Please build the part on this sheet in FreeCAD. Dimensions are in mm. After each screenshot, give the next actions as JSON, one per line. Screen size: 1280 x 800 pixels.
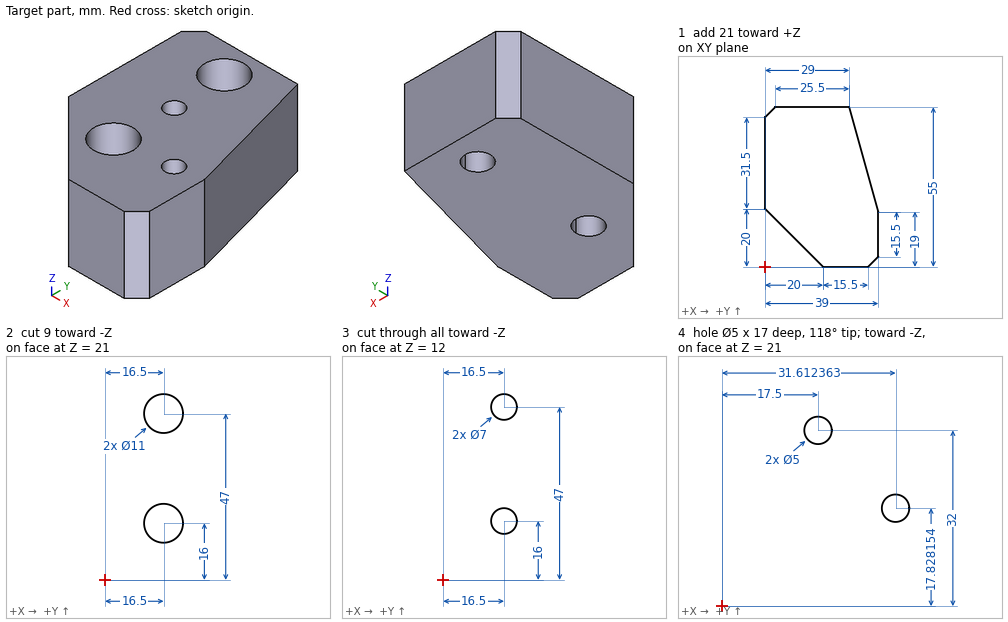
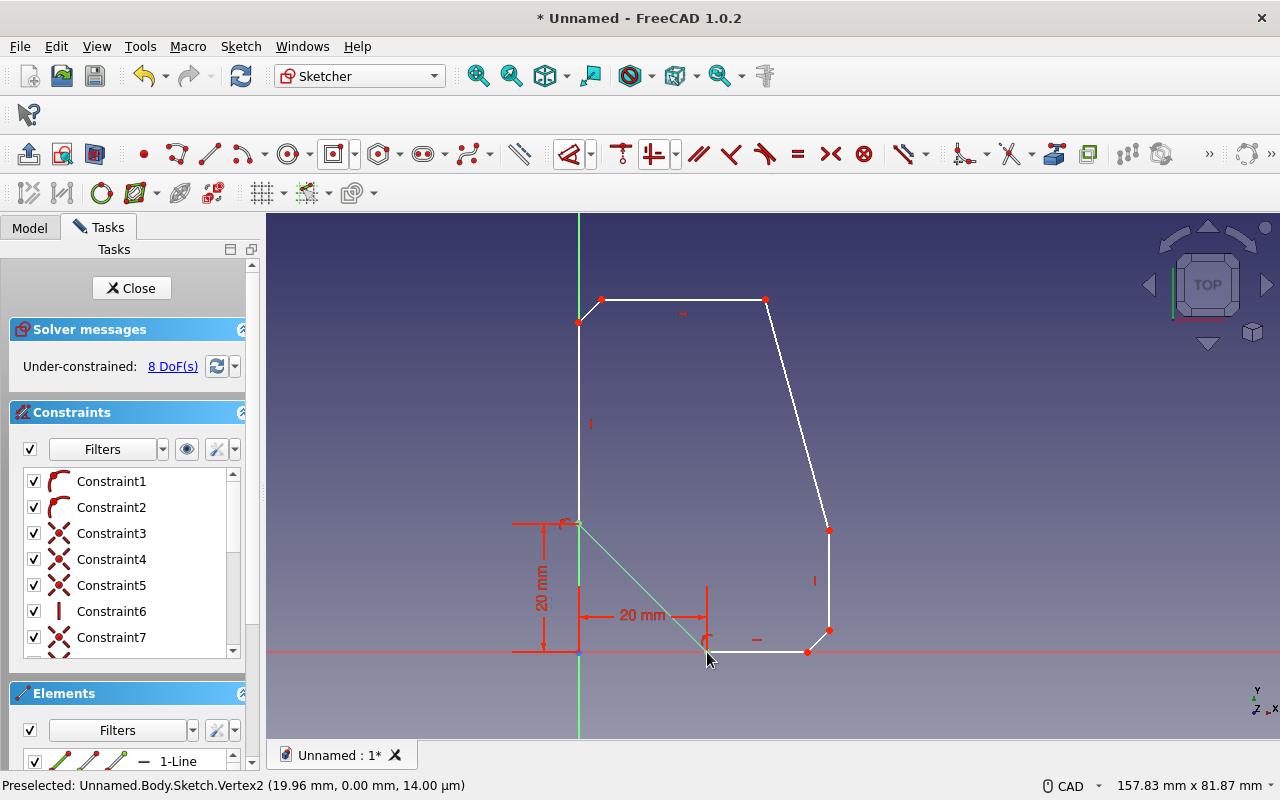
{"action": "left_click", "coordinate": [829, 631]}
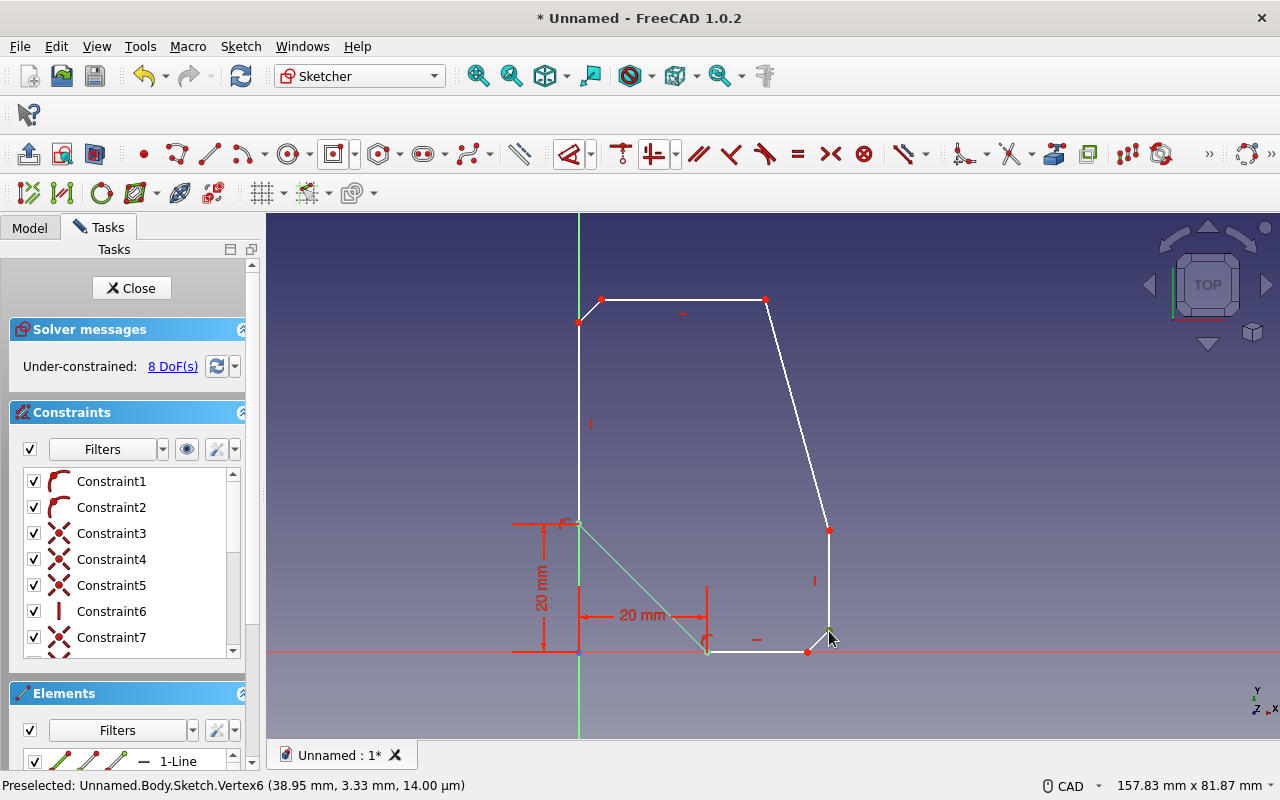
{"action": "key", "text": "l"}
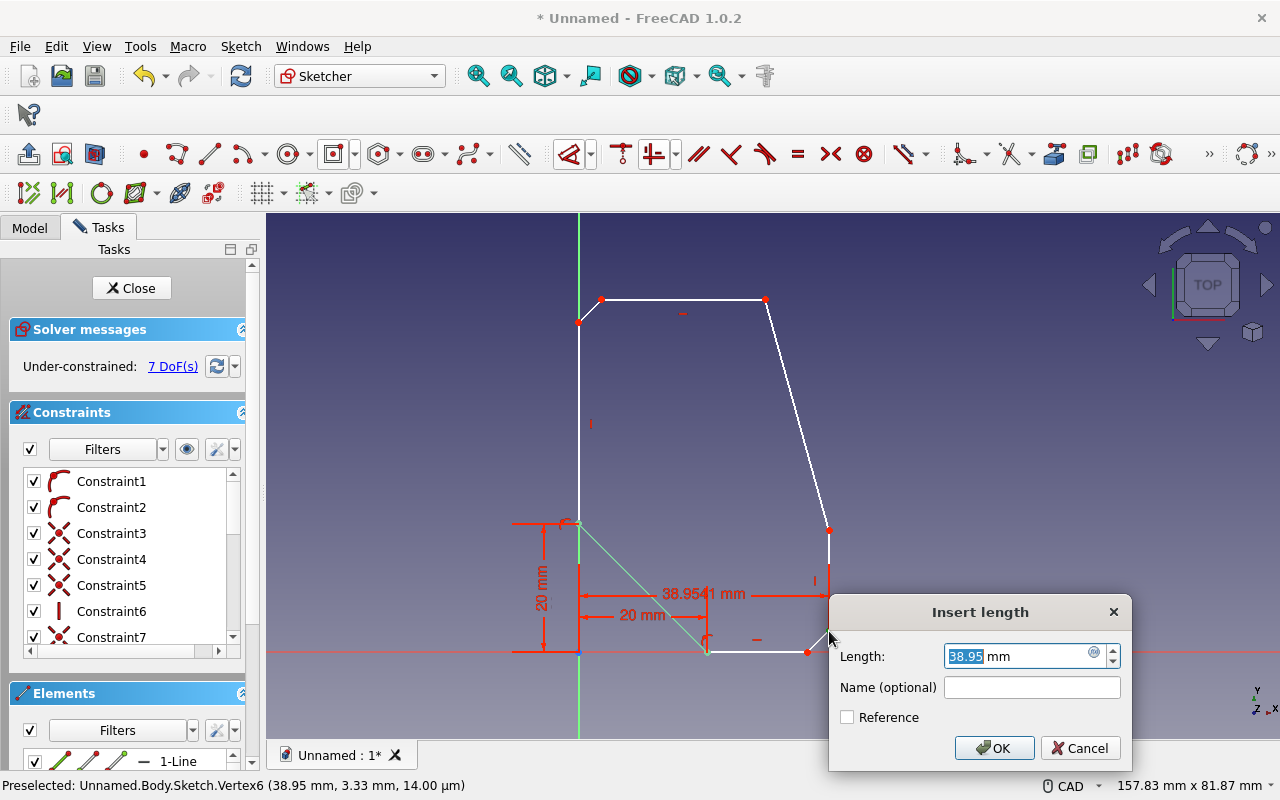
{"action": "type", "text": "39"}
{"action": "key", "text": "Return"}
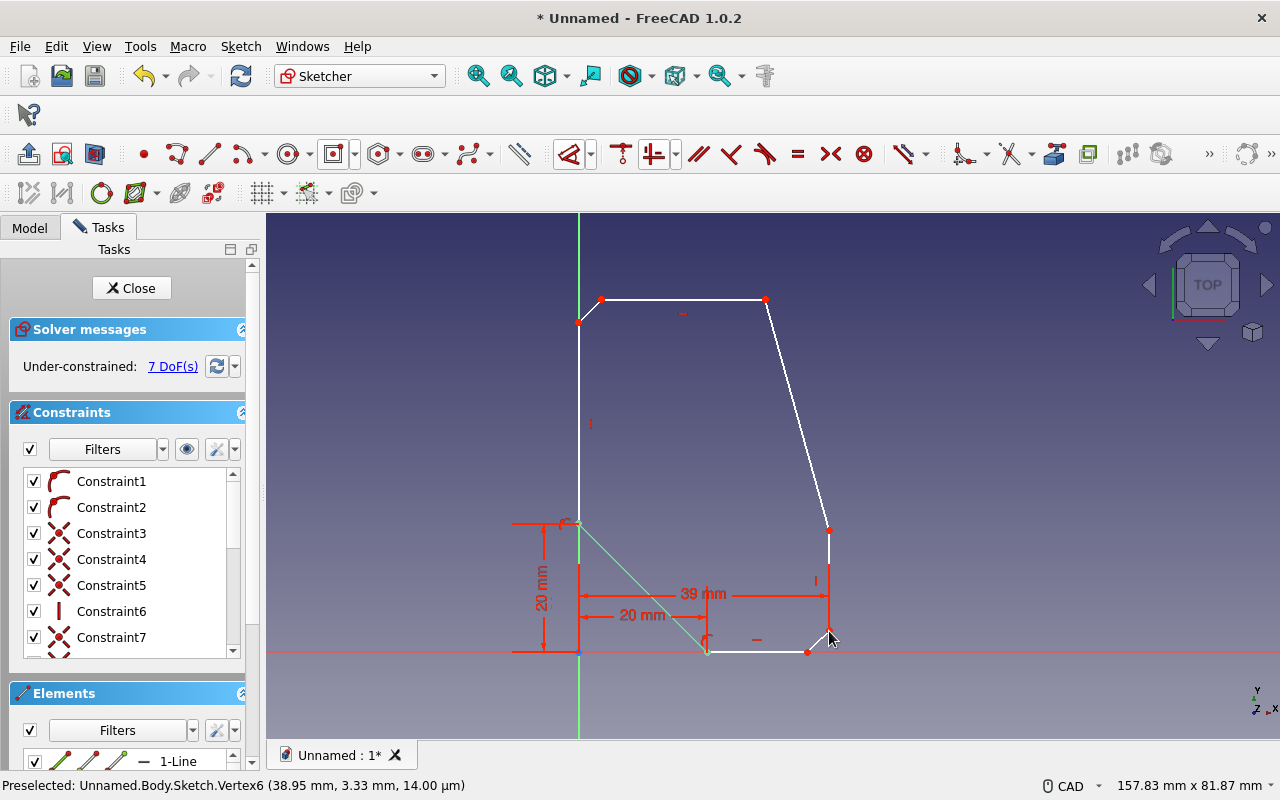
{"action": "left_click", "coordinate": [829, 531]}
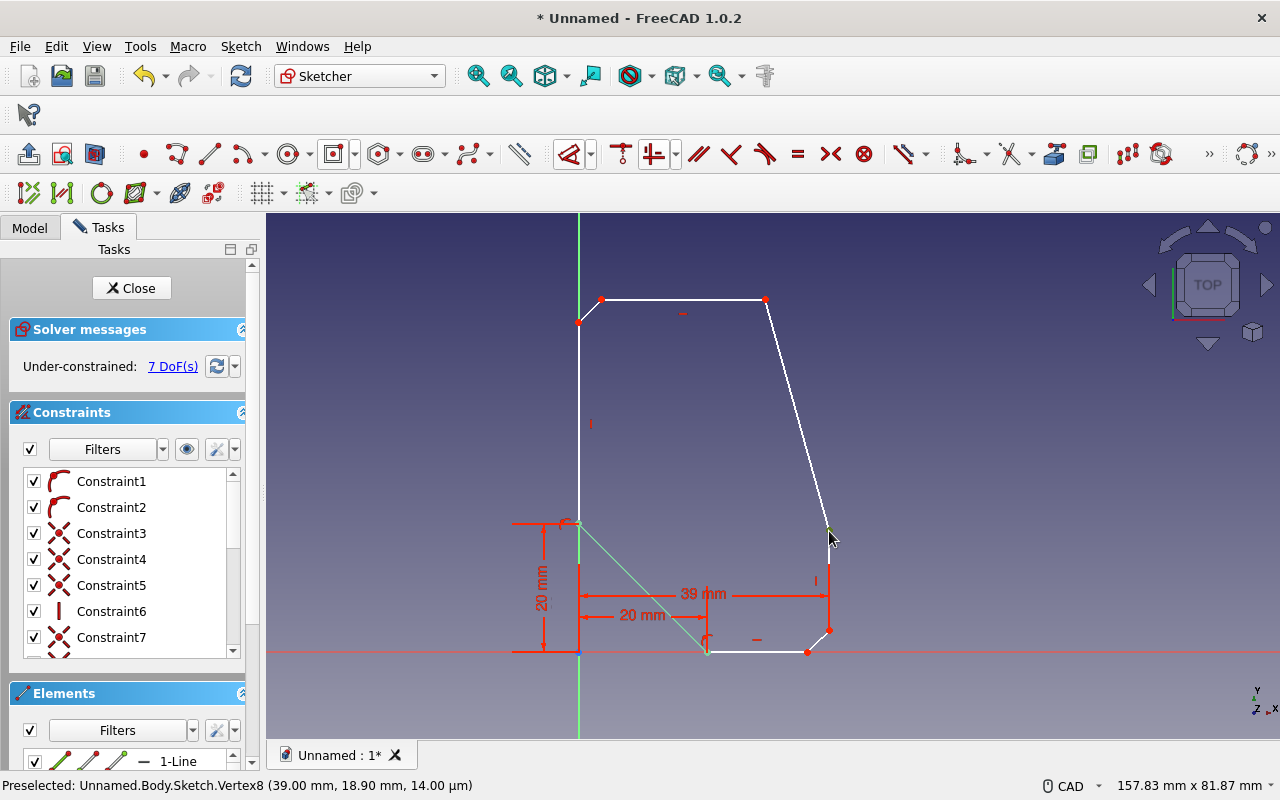
{"action": "key", "text": "i"}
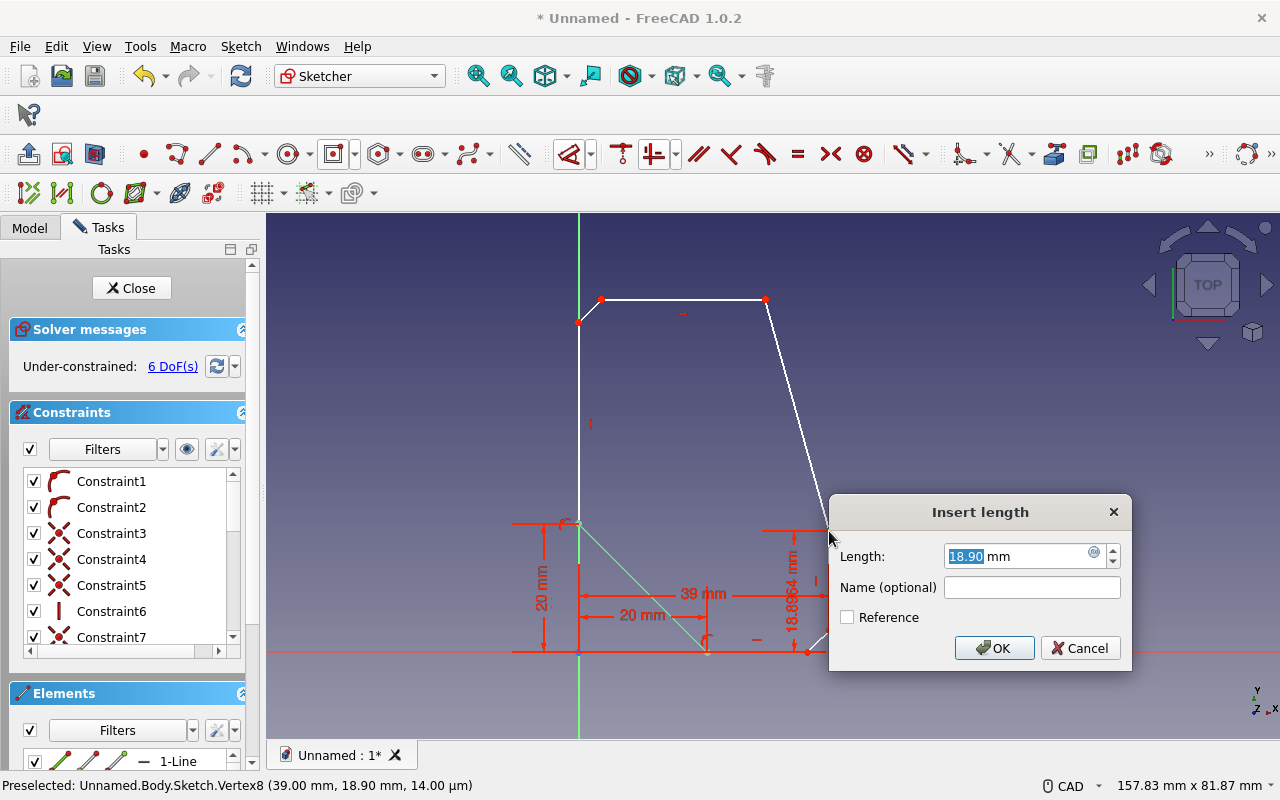
{"action": "type", "text": "19"}
{"action": "key", "text": "Return"}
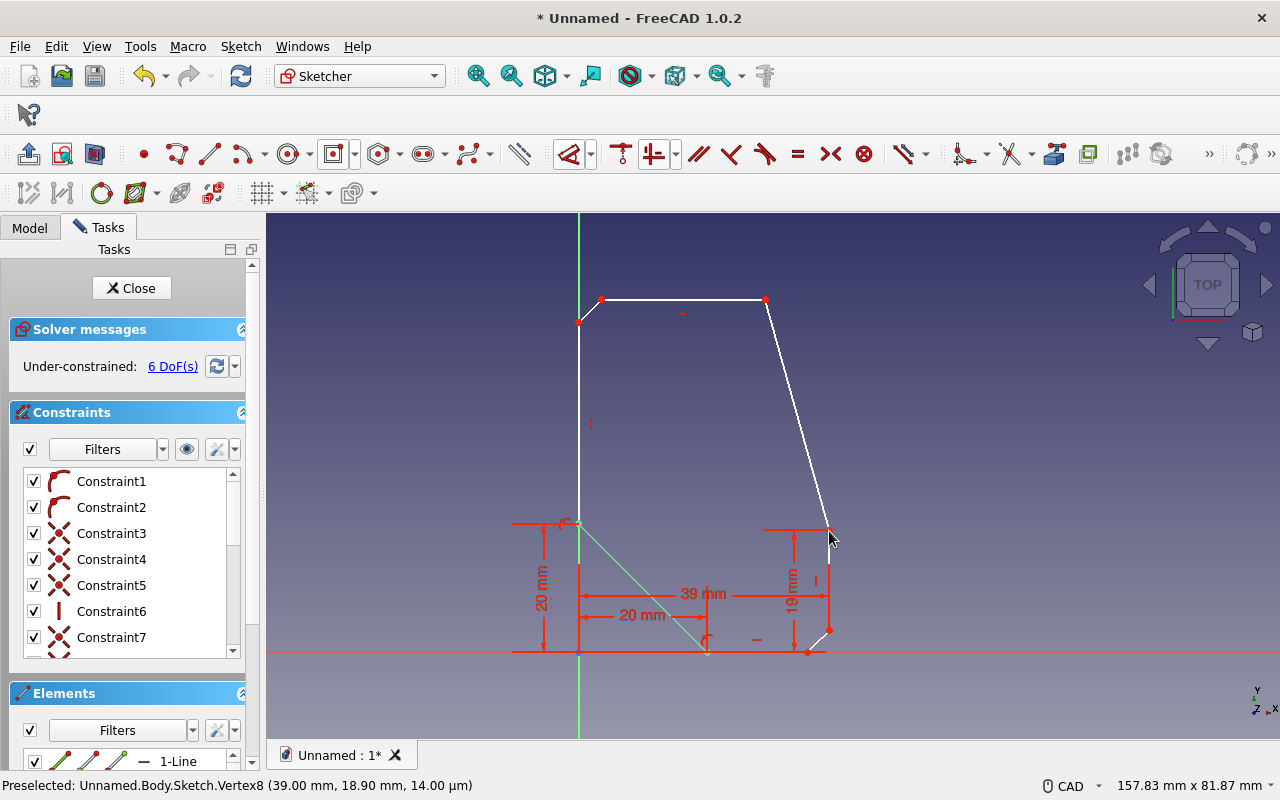
{"action": "left_click", "coordinate": [765, 300]}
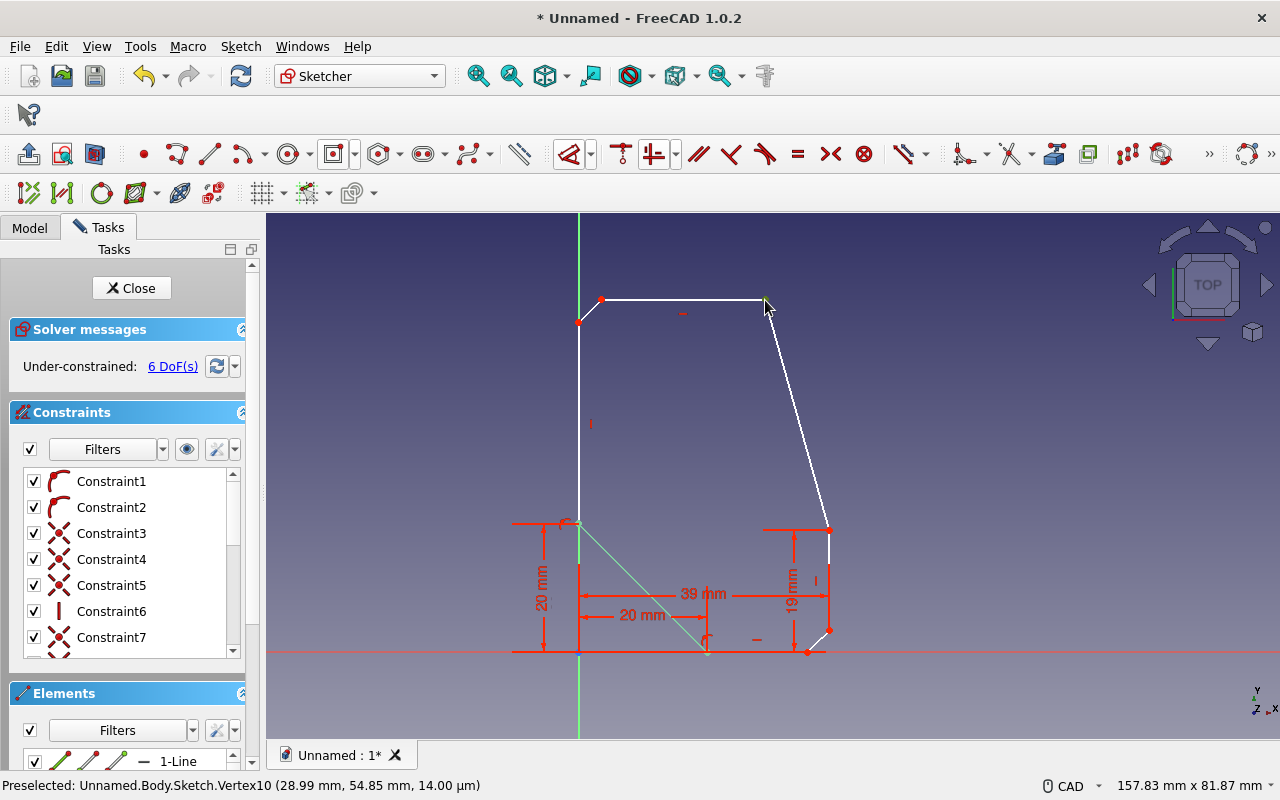
{"action": "key", "text": "l"}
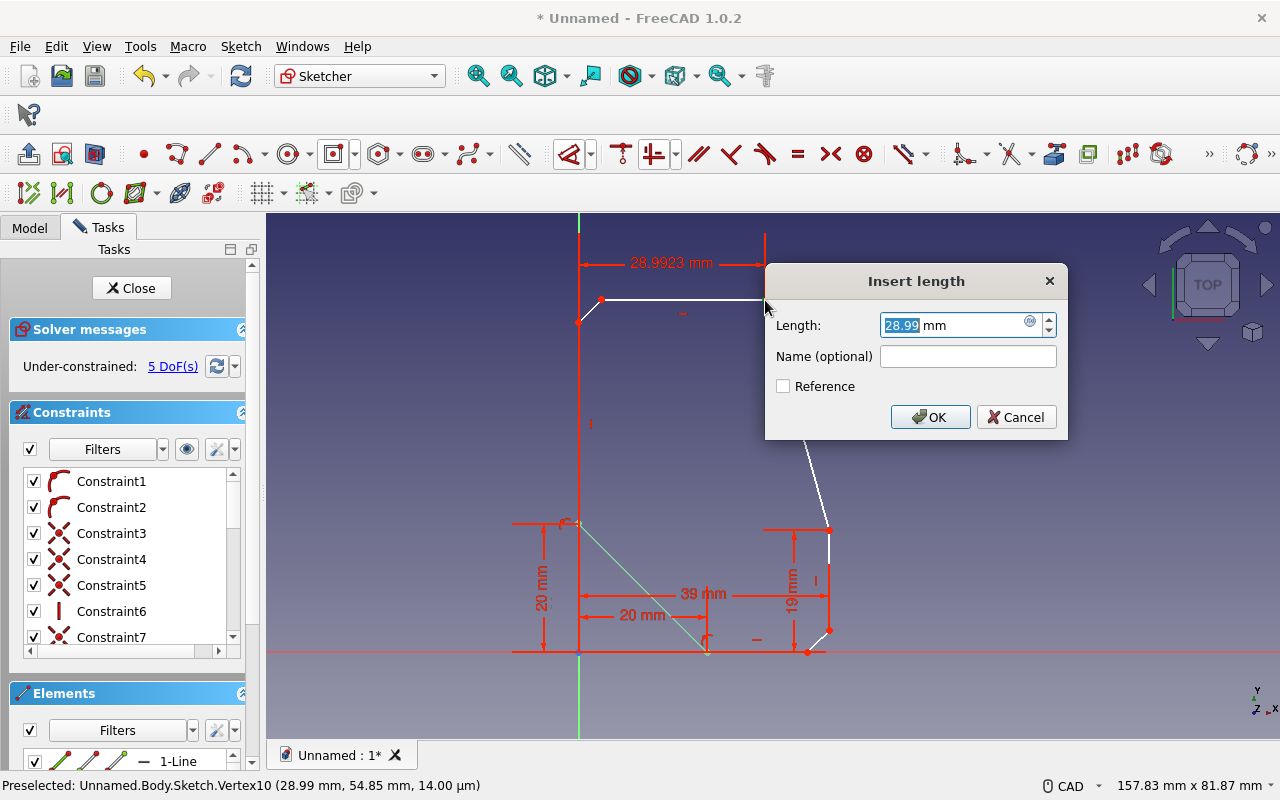
{"action": "type", "text": "29"}
{"action": "key", "text": "Return"}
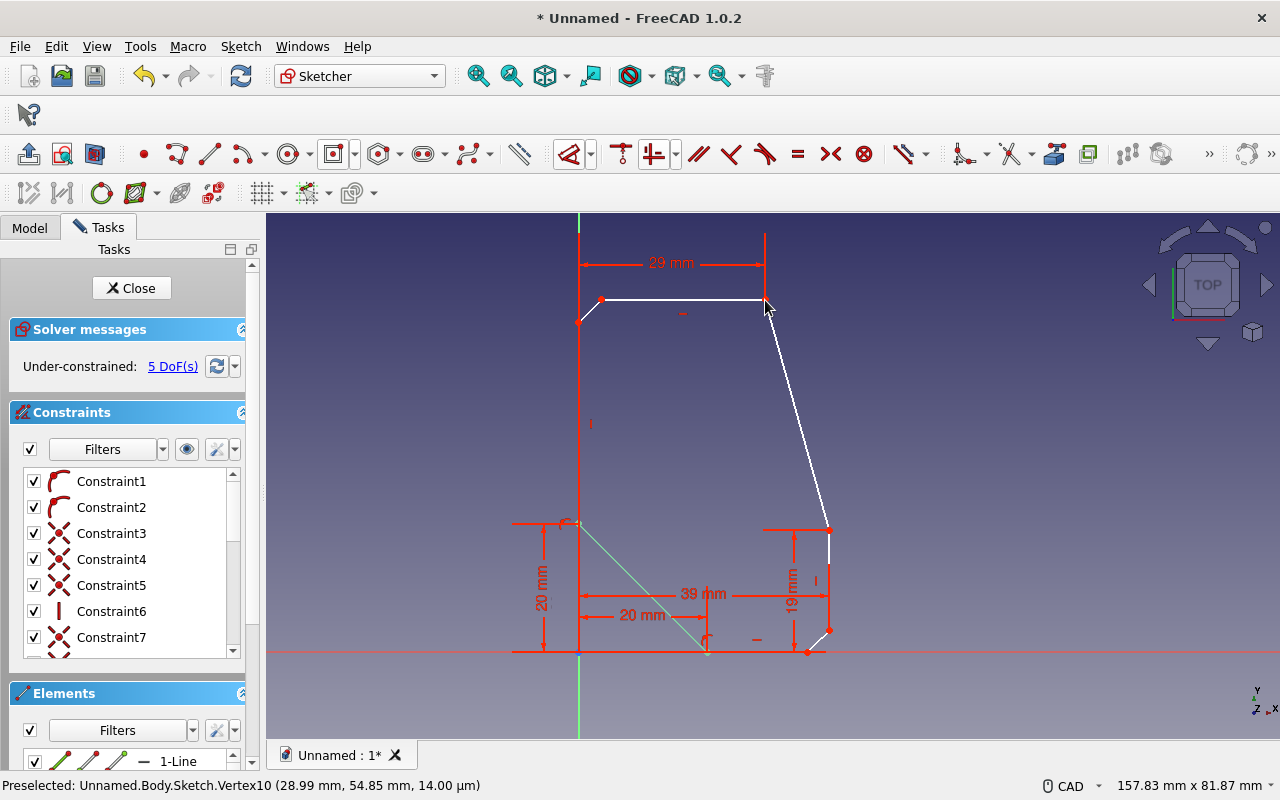
{"action": "left_click", "coordinate": [765, 300]}